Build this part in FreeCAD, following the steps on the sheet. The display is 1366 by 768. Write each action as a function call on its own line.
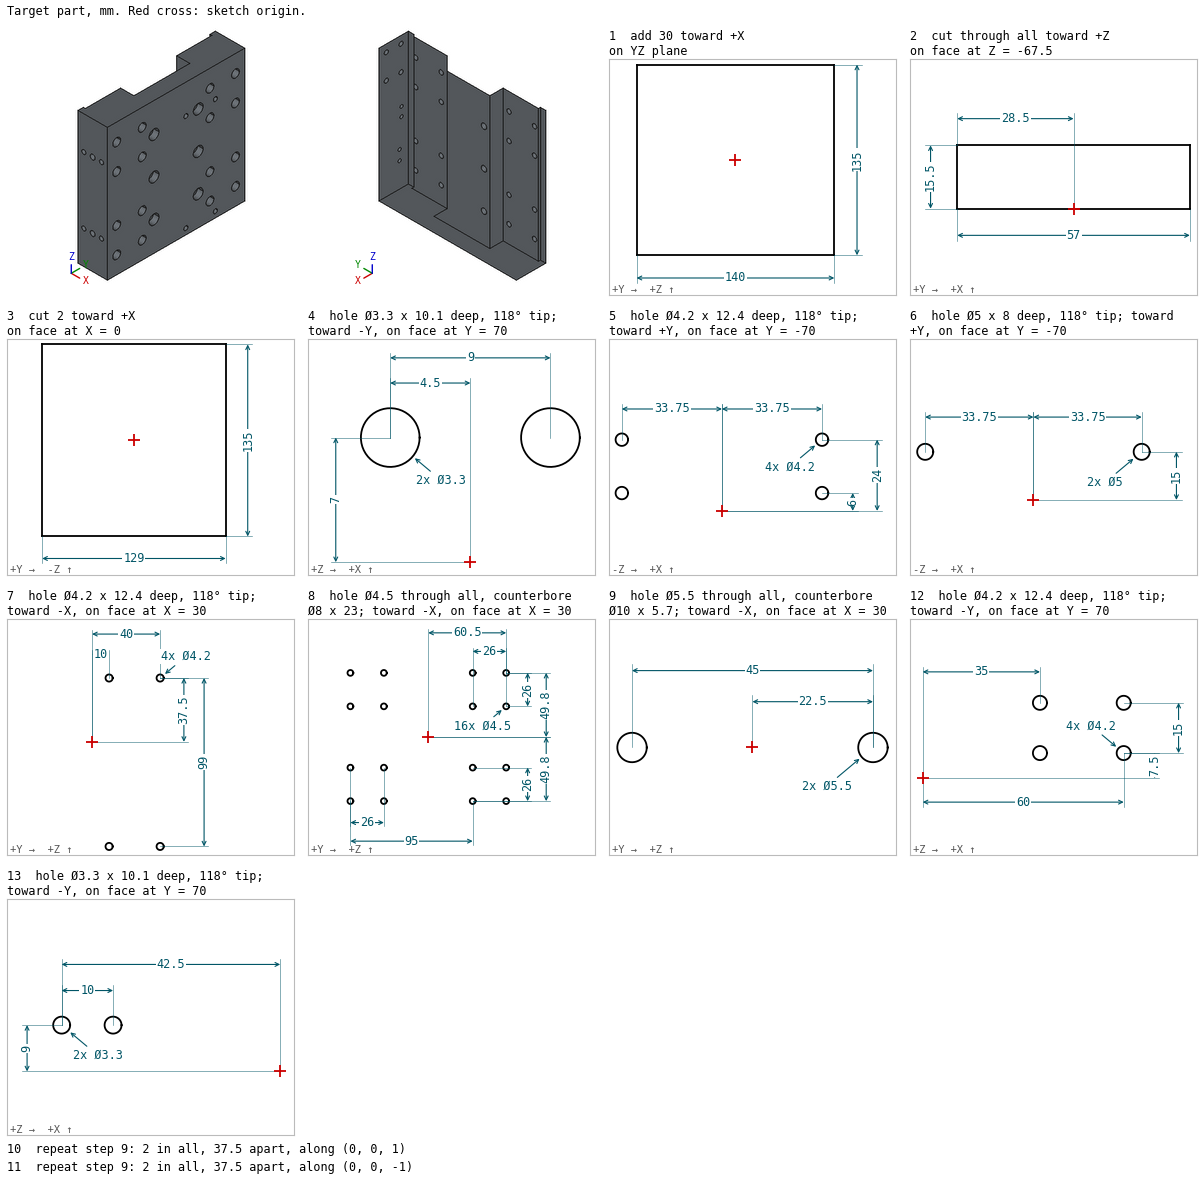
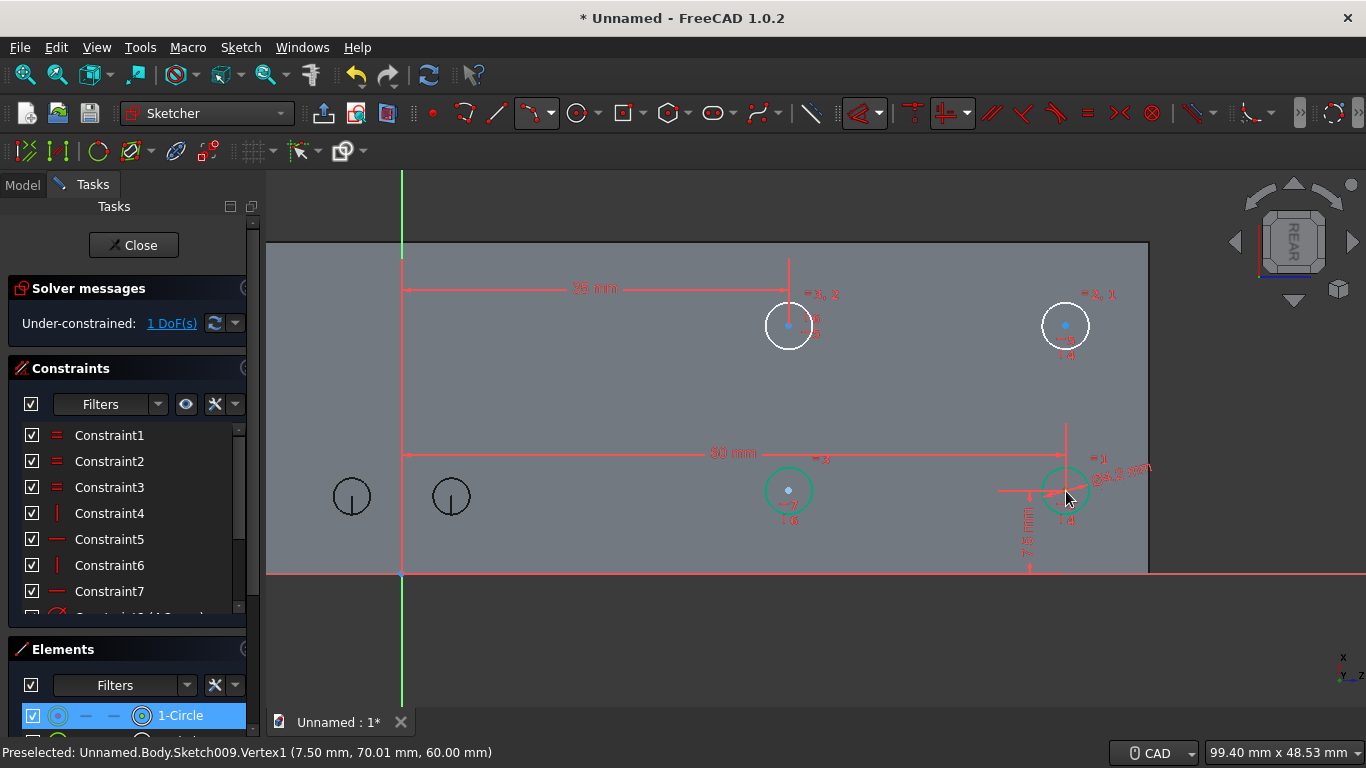
click(1066, 326)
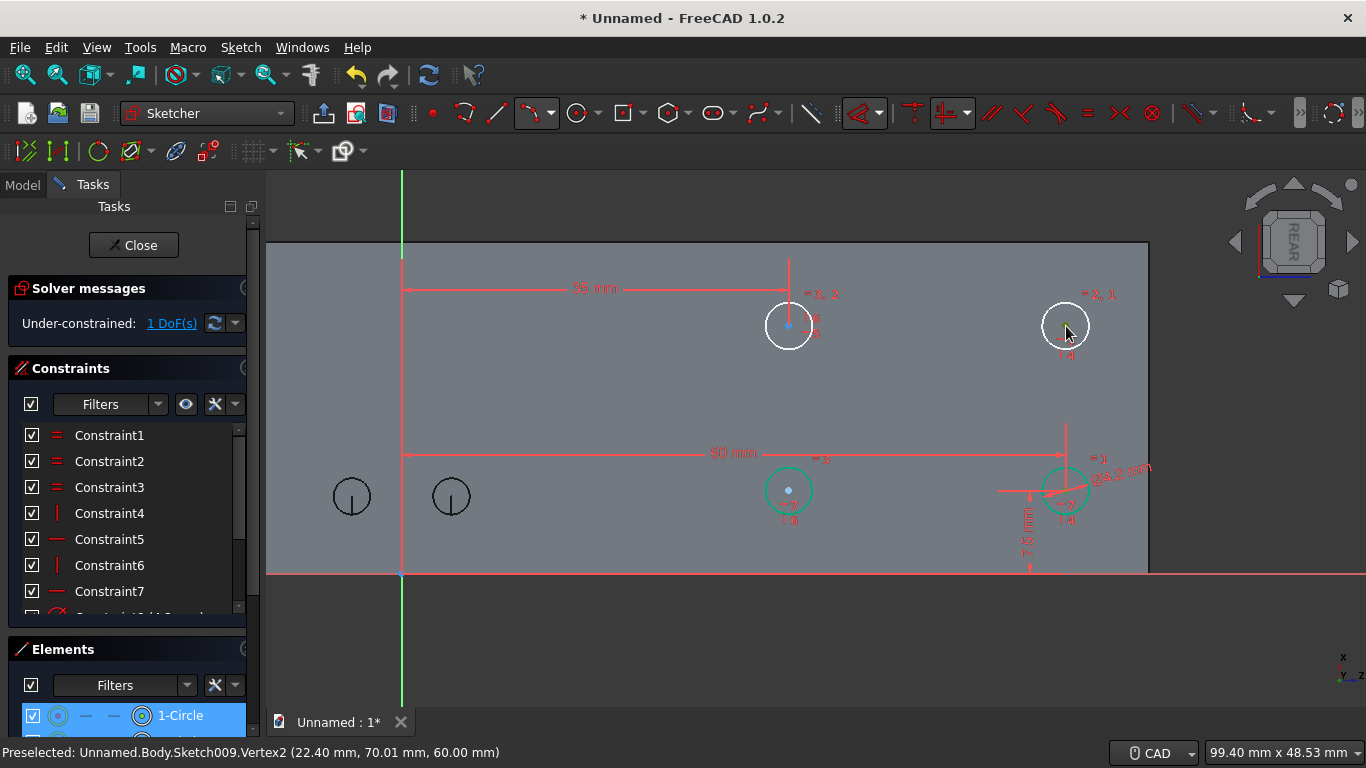
click(882, 114)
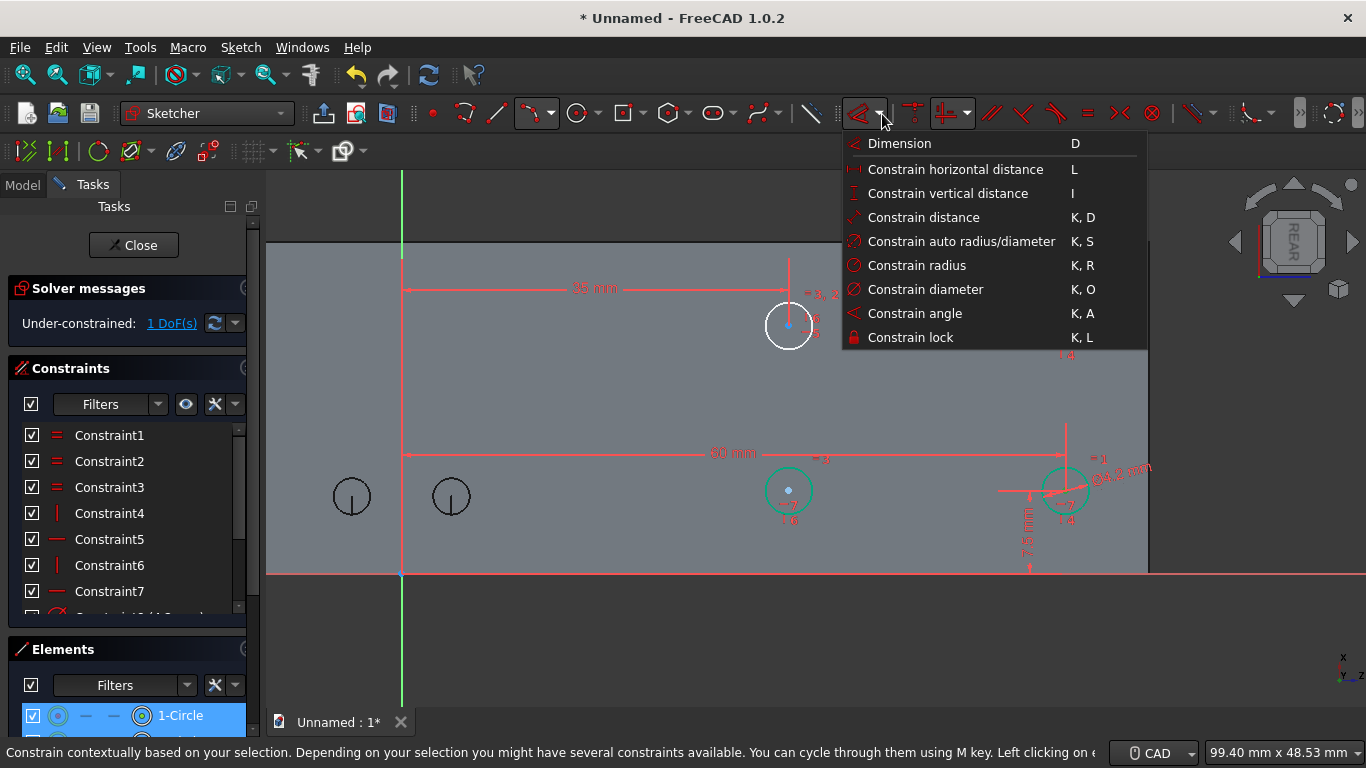
click(995, 193)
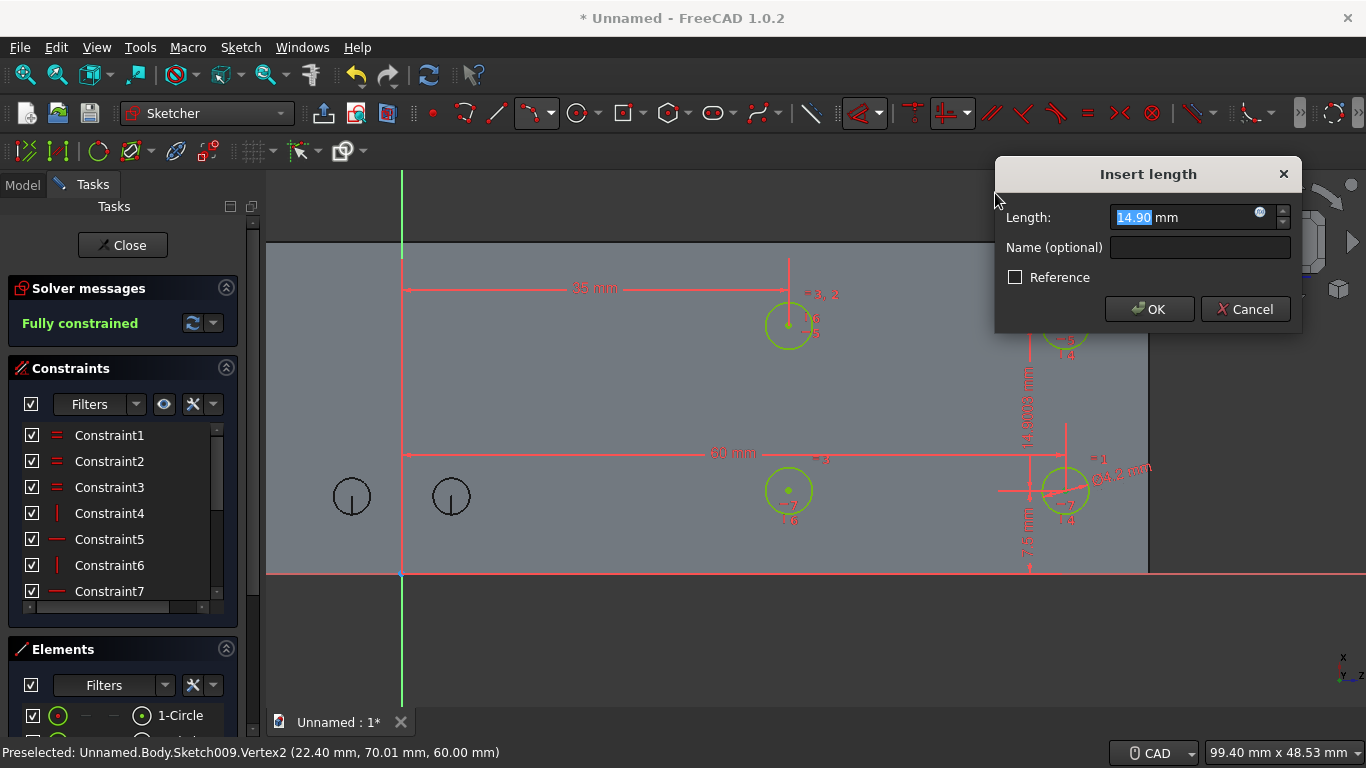
text(15)
key(Return)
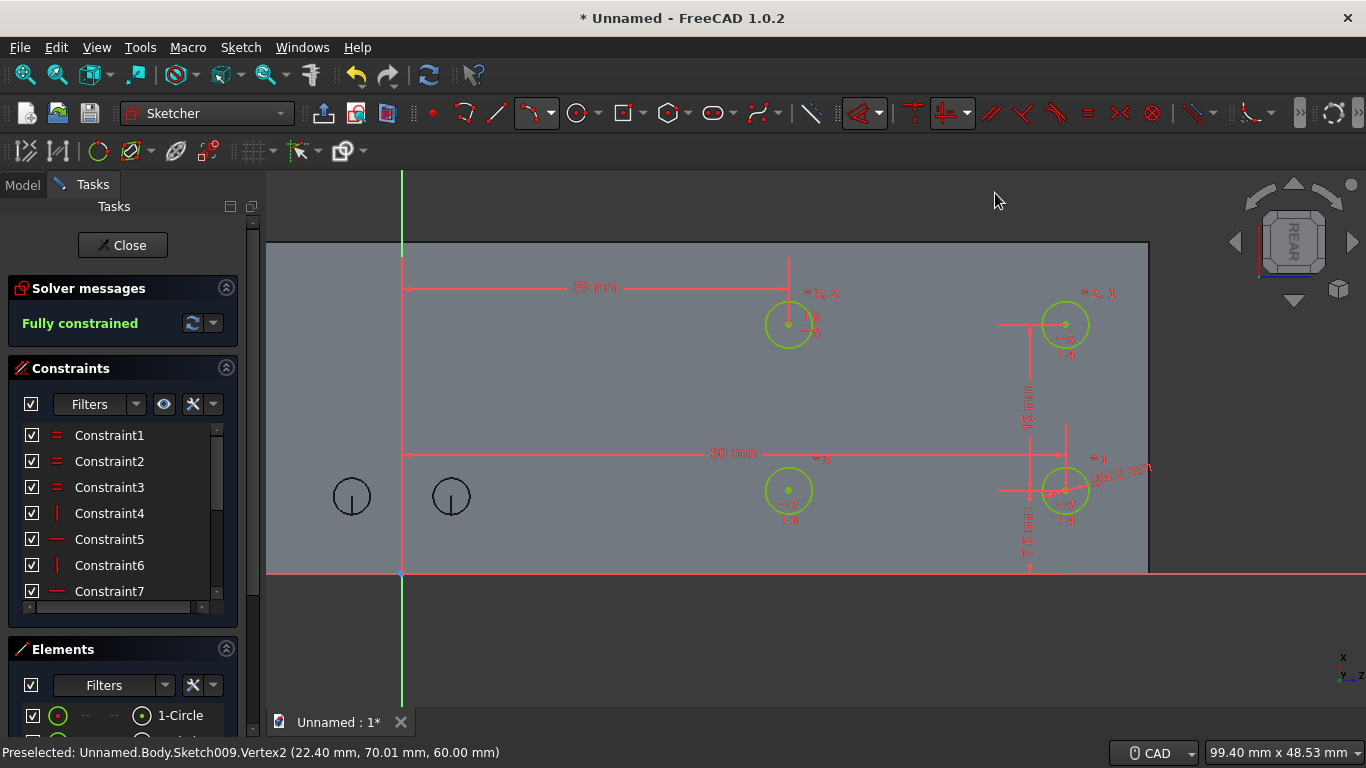
click(123, 245)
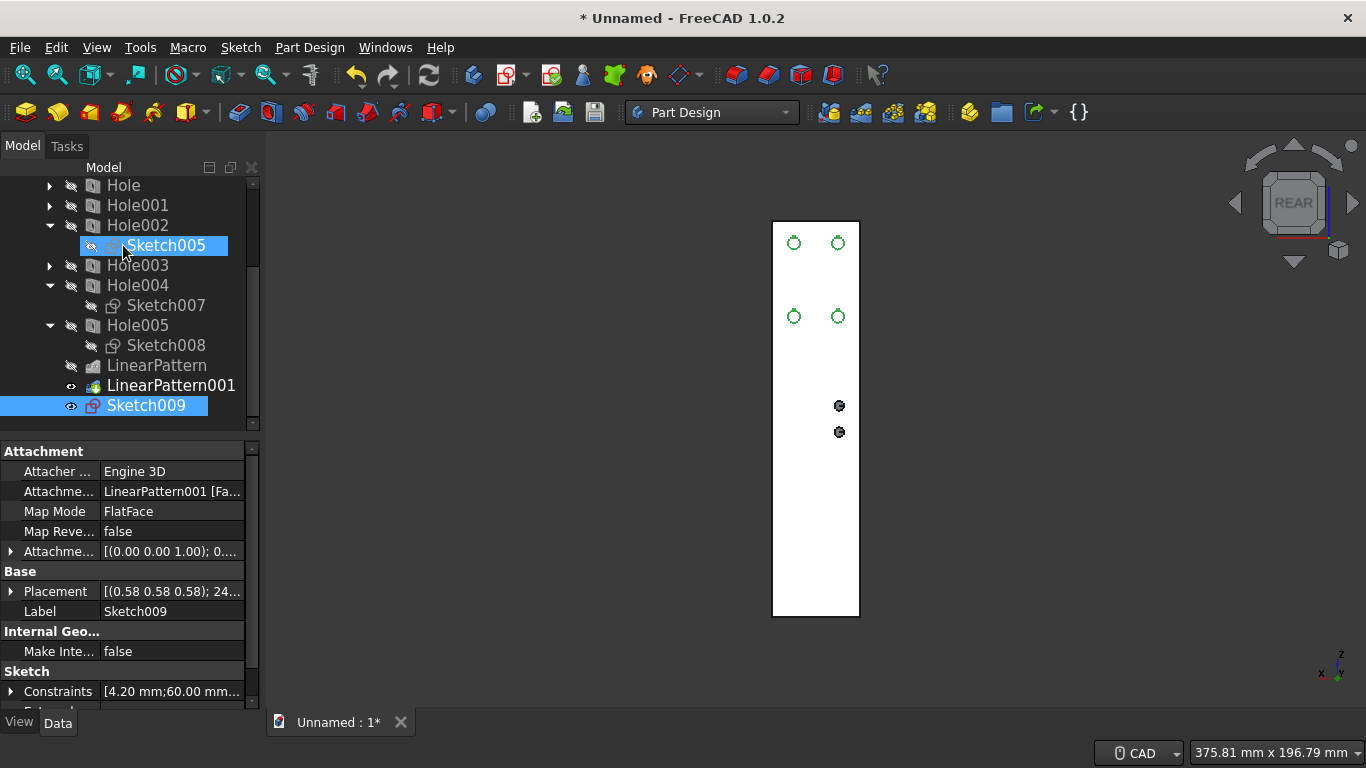
click(272, 112)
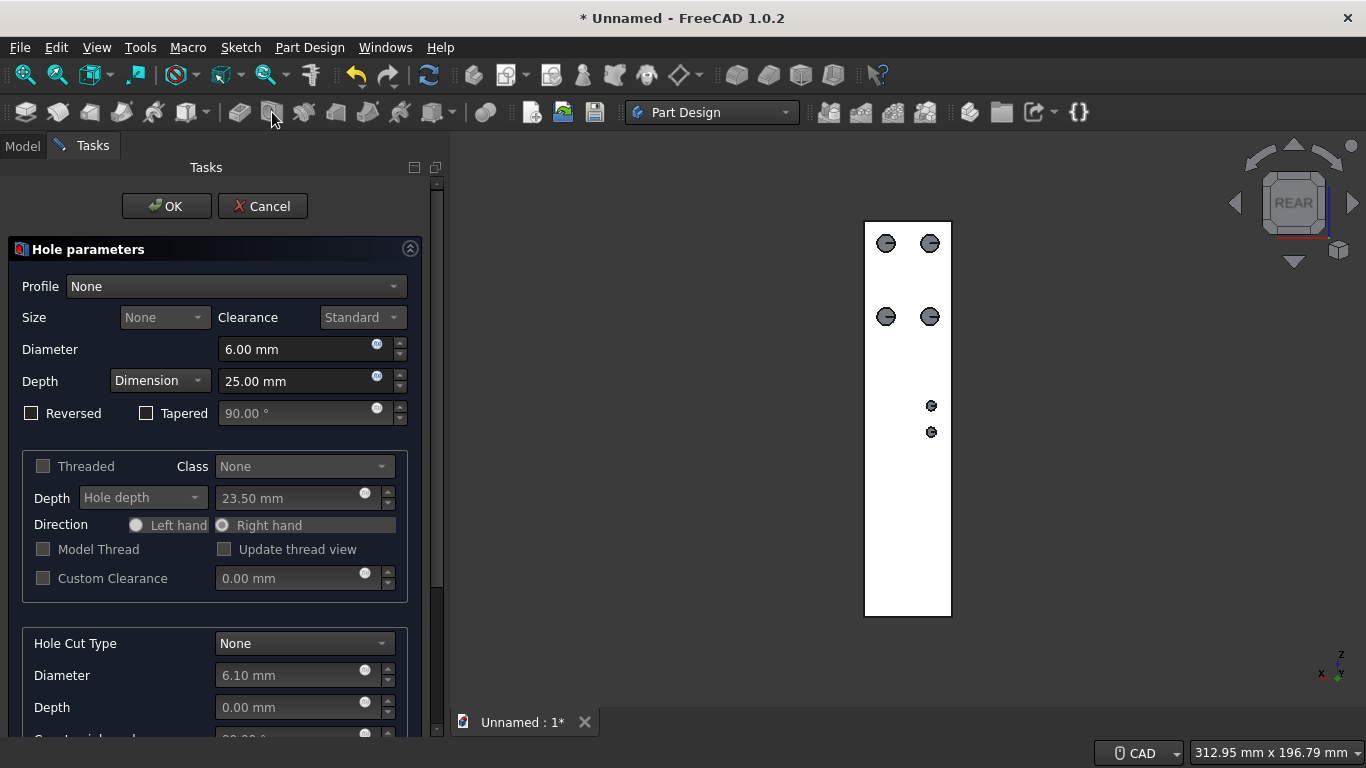
triple_click(305, 349)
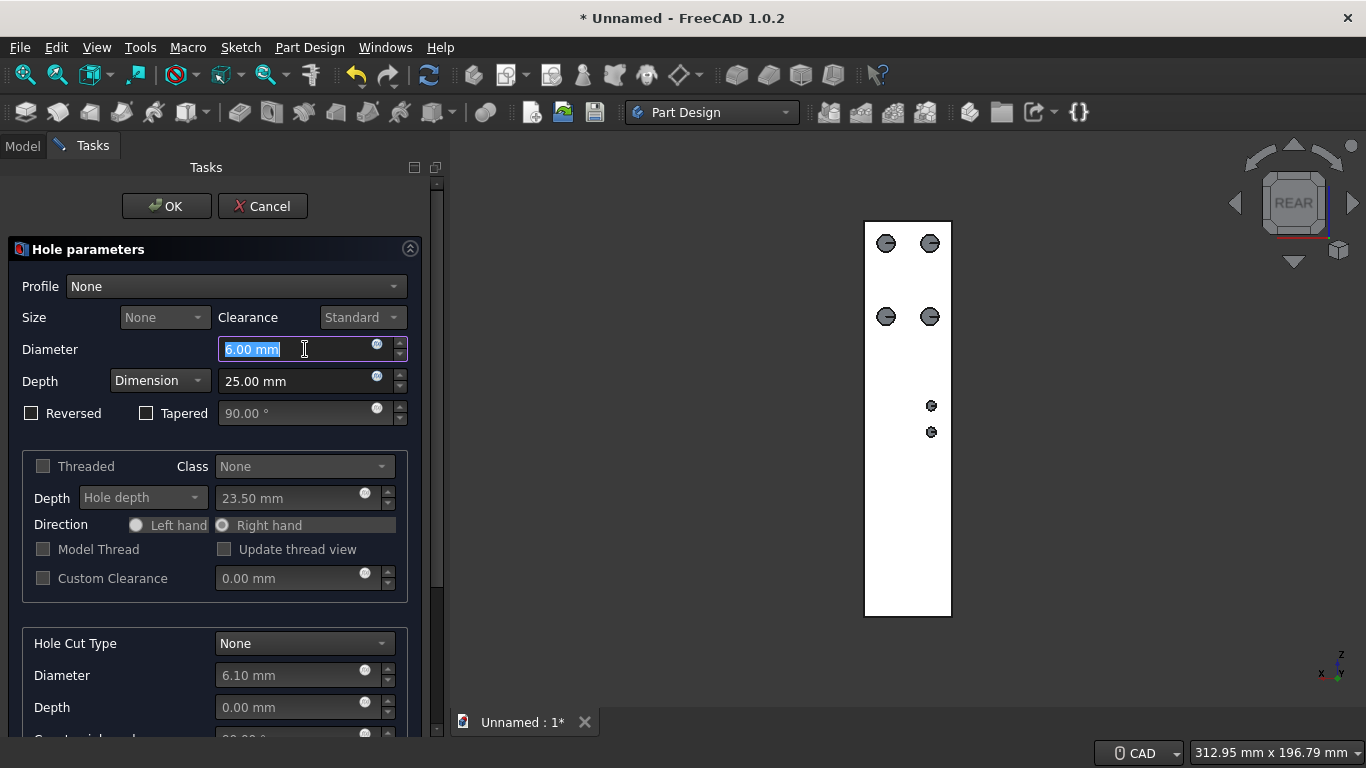
text(4.2)
key(Tab)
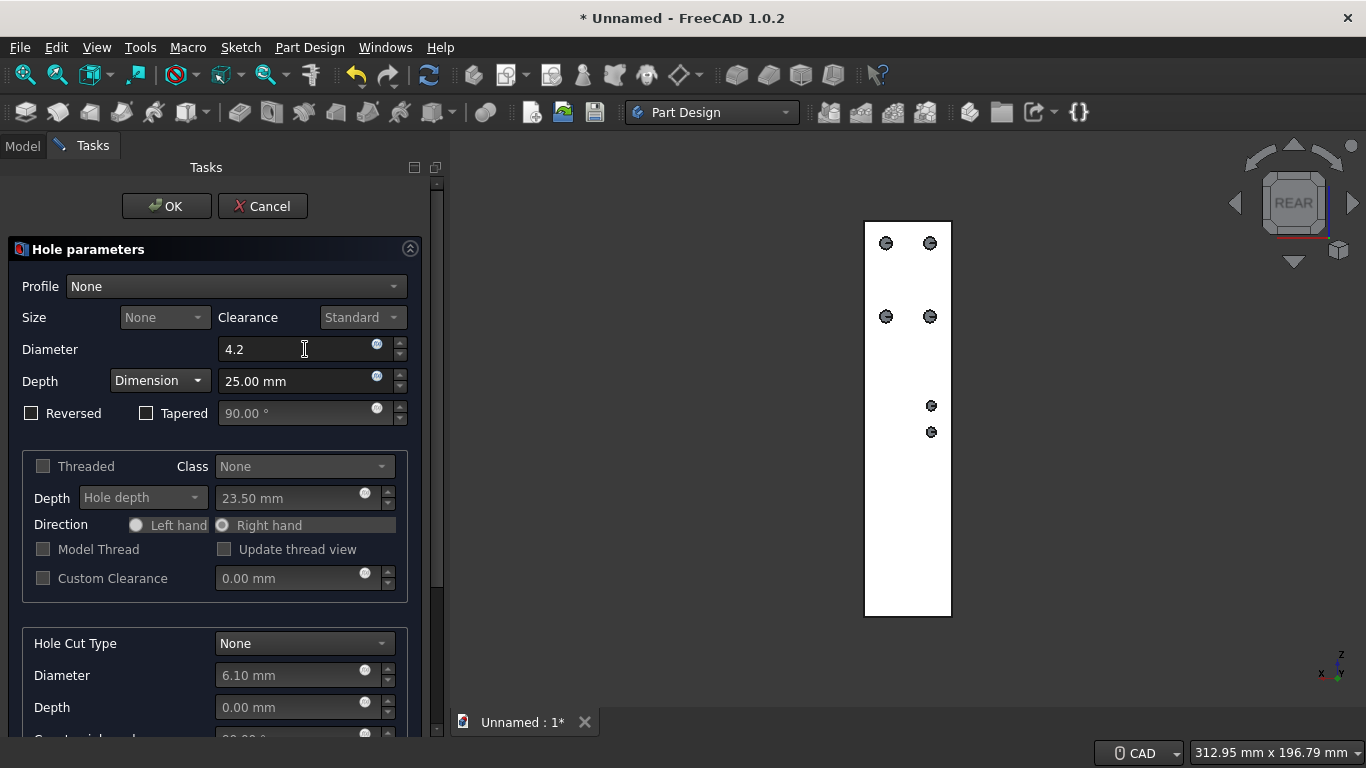
triple_click(305, 381)